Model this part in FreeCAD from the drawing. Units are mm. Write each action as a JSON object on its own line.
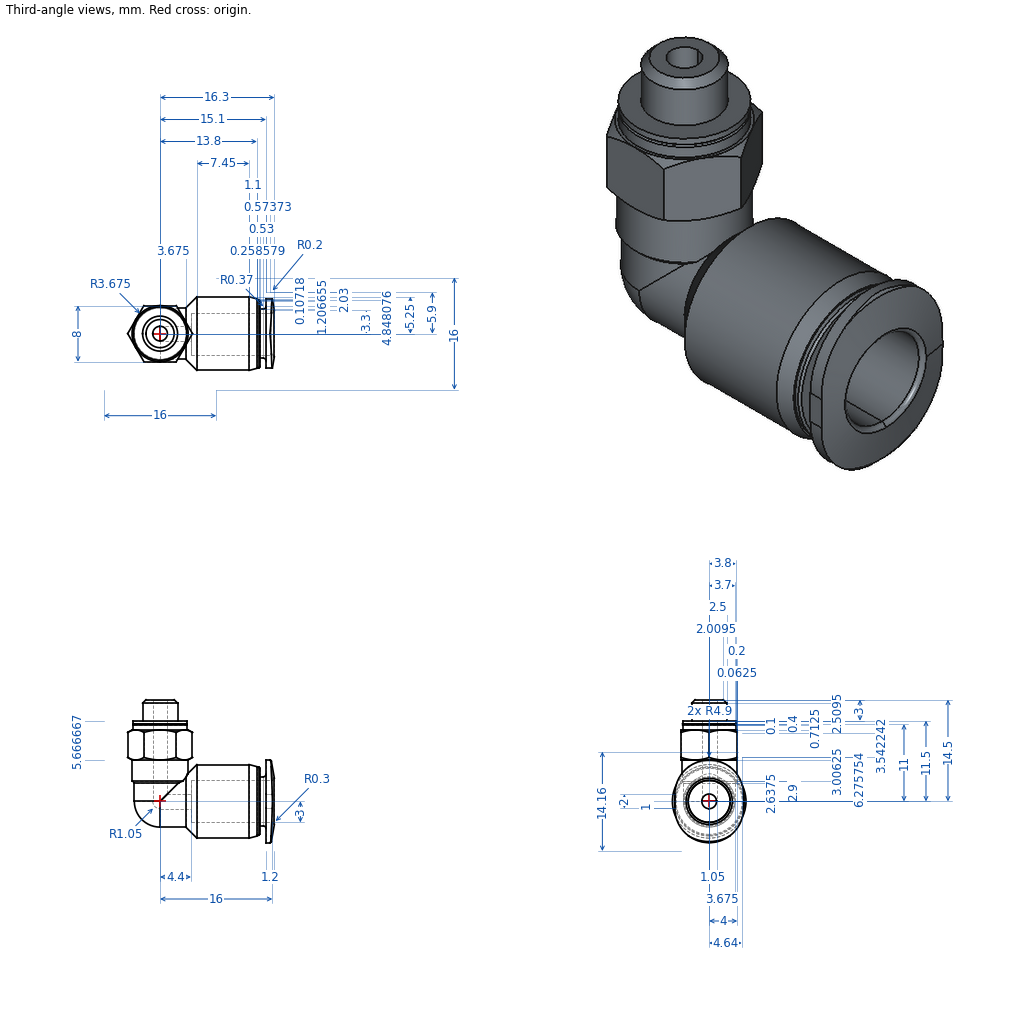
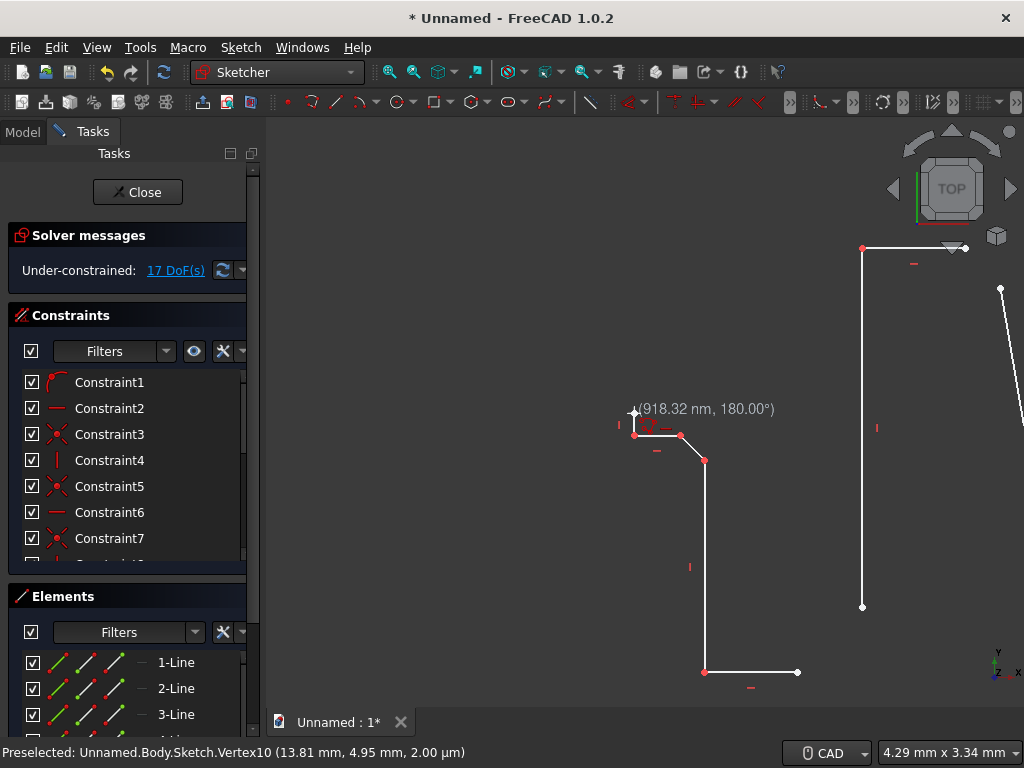
{"action": "scroll", "coordinate": [734, 368], "scroll_direction": "down", "scroll_amount": 11}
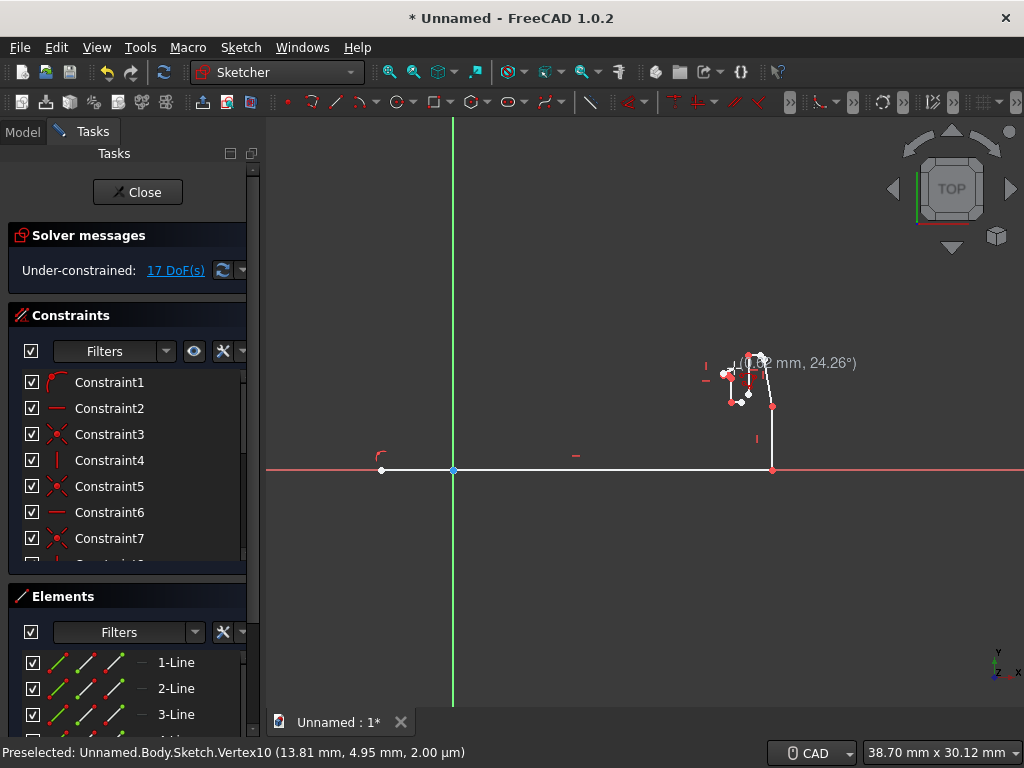
{"action": "left_click", "coordinate": [702, 368]}
{"action": "left_click", "coordinate": [556, 368]}
{"action": "left_click", "coordinate": [525, 398]}
{"action": "left_click", "coordinate": [453, 398]}
{"action": "right_click", "coordinate": [453, 398]}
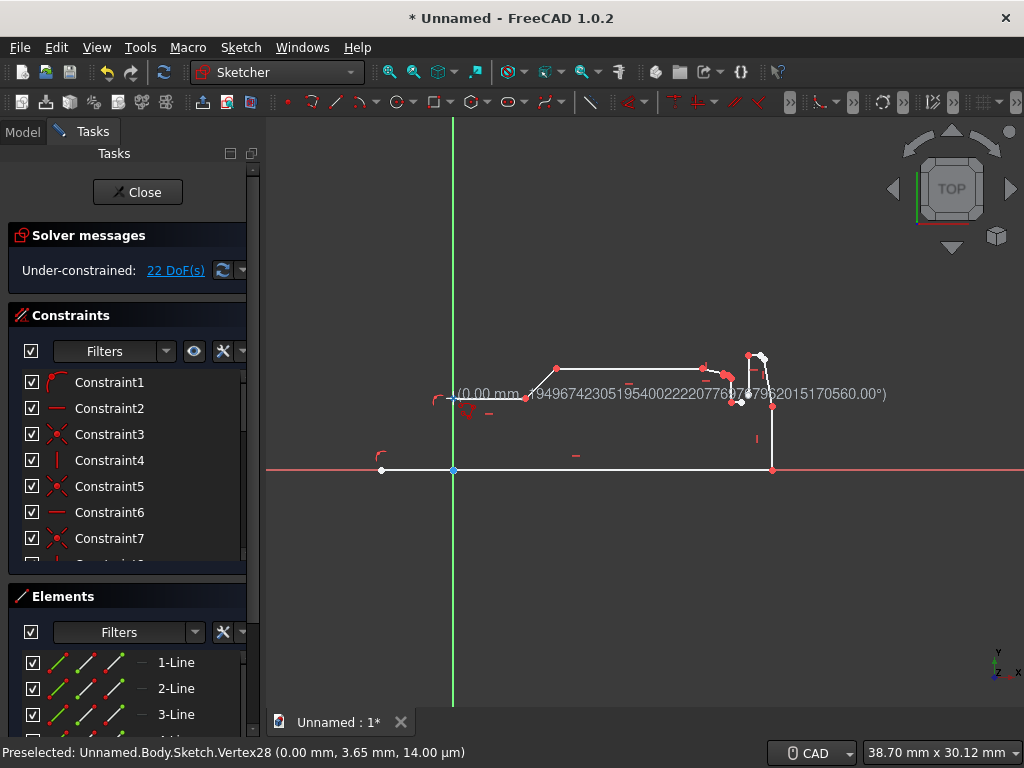
{"action": "key", "text": "g 3 a"}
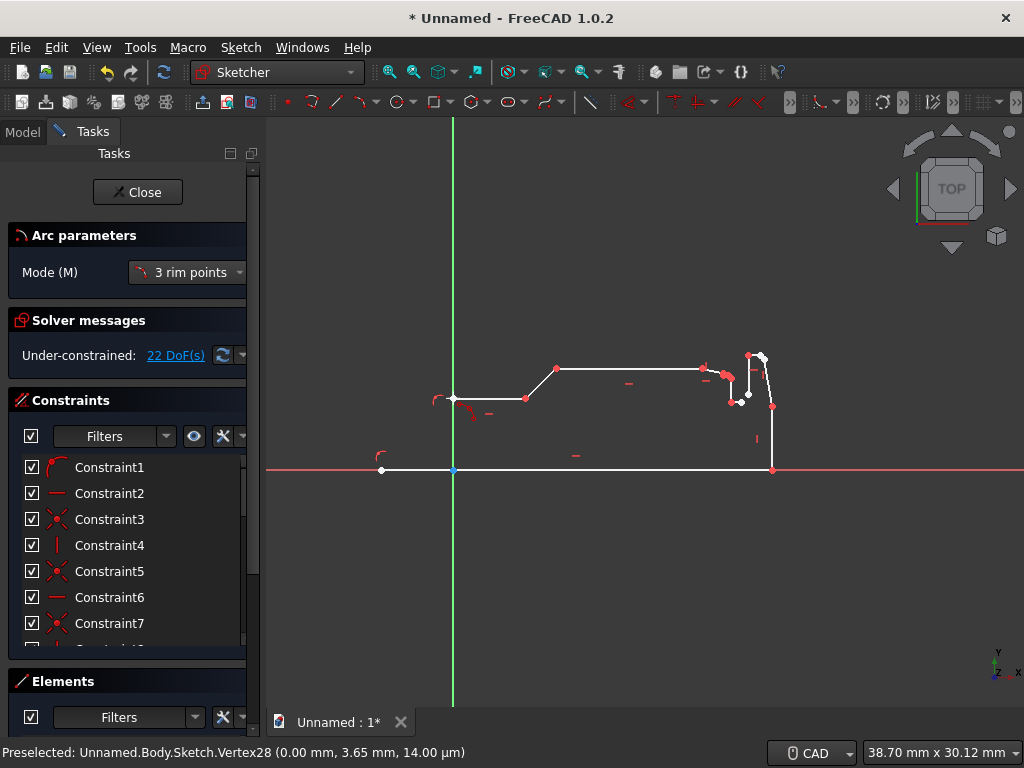
{"action": "scroll", "coordinate": [764, 358], "scroll_direction": "up", "scroll_amount": 6}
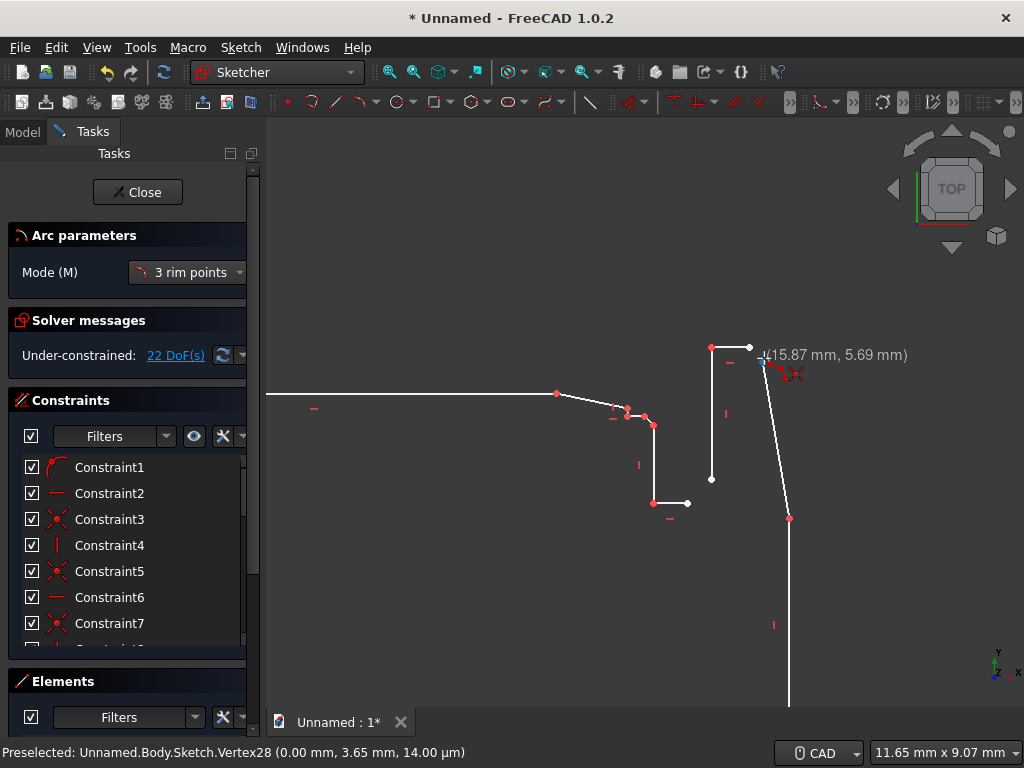
{"action": "left_click", "coordinate": [763, 362]}
{"action": "left_click", "coordinate": [750, 347]}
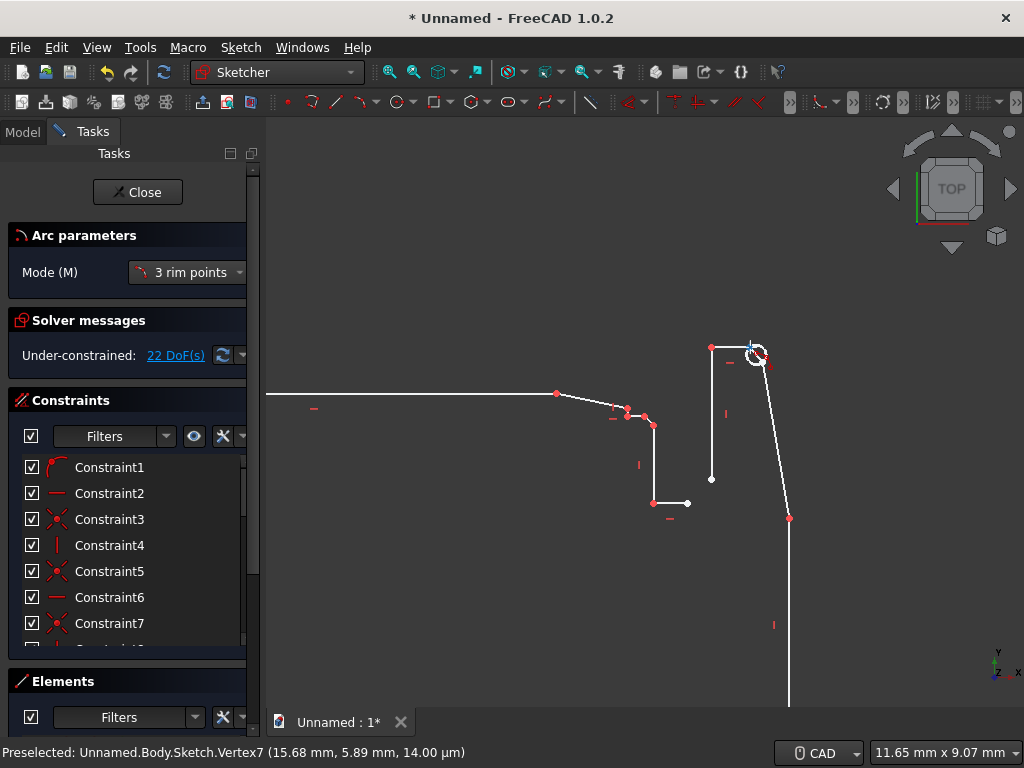
{"action": "scroll", "coordinate": [758, 350], "scroll_direction": "up", "scroll_amount": 9}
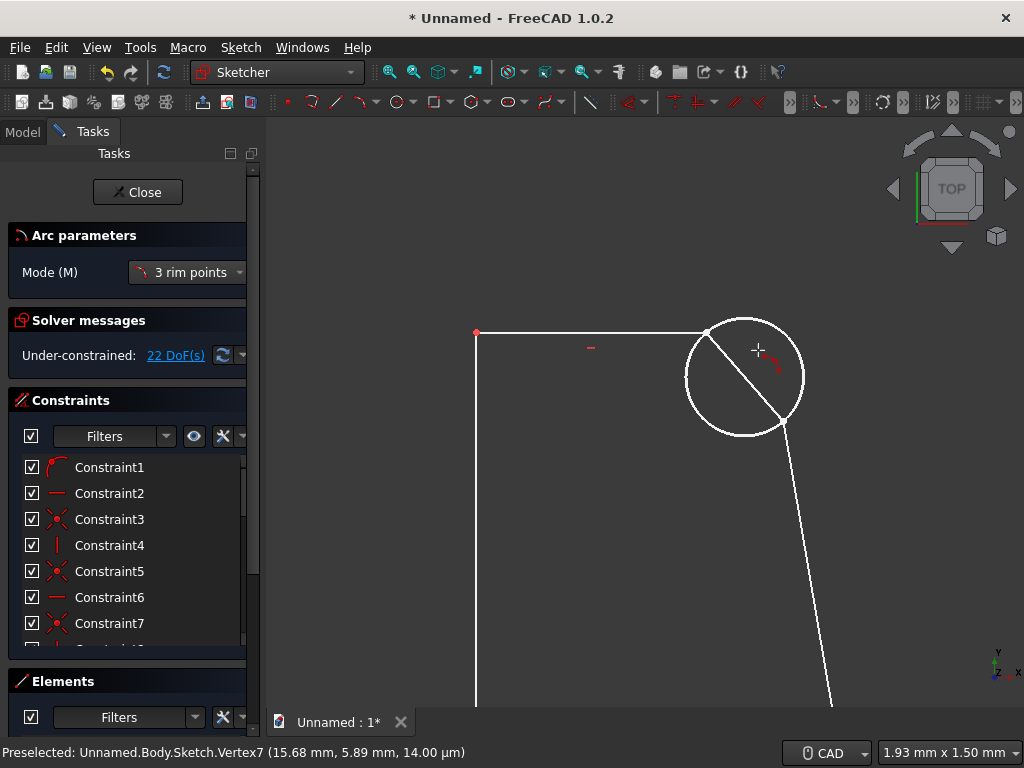
{"action": "left_click", "coordinate": [754, 347]}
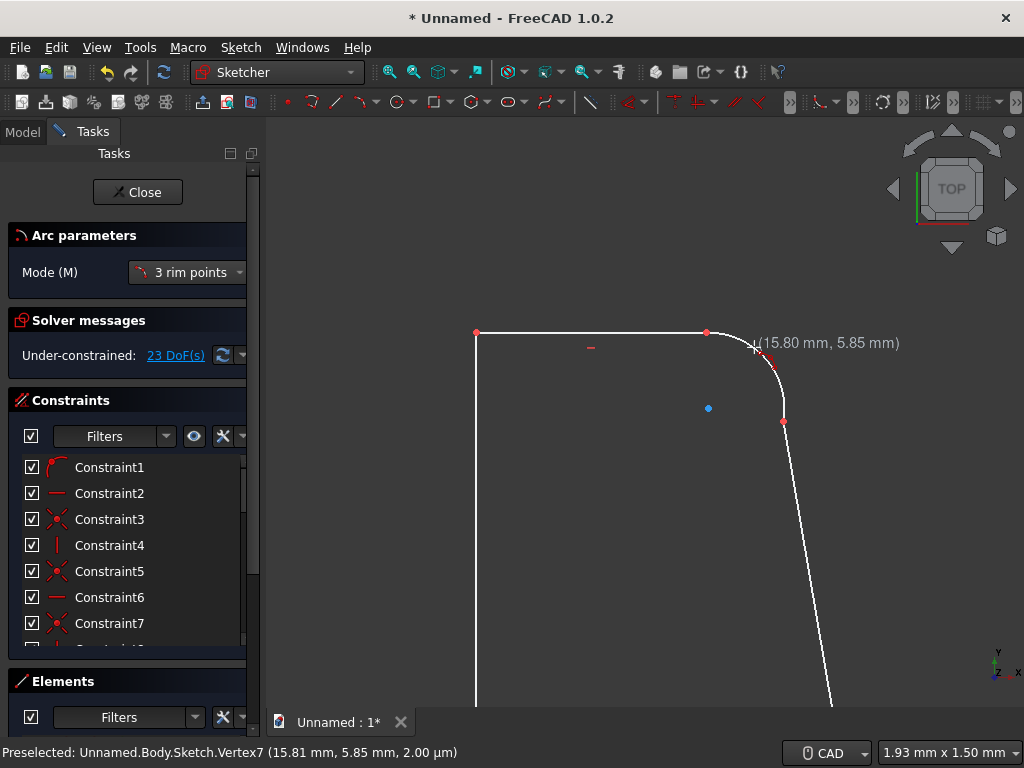
{"action": "scroll", "coordinate": [763, 356], "scroll_direction": "down", "scroll_amount": 15}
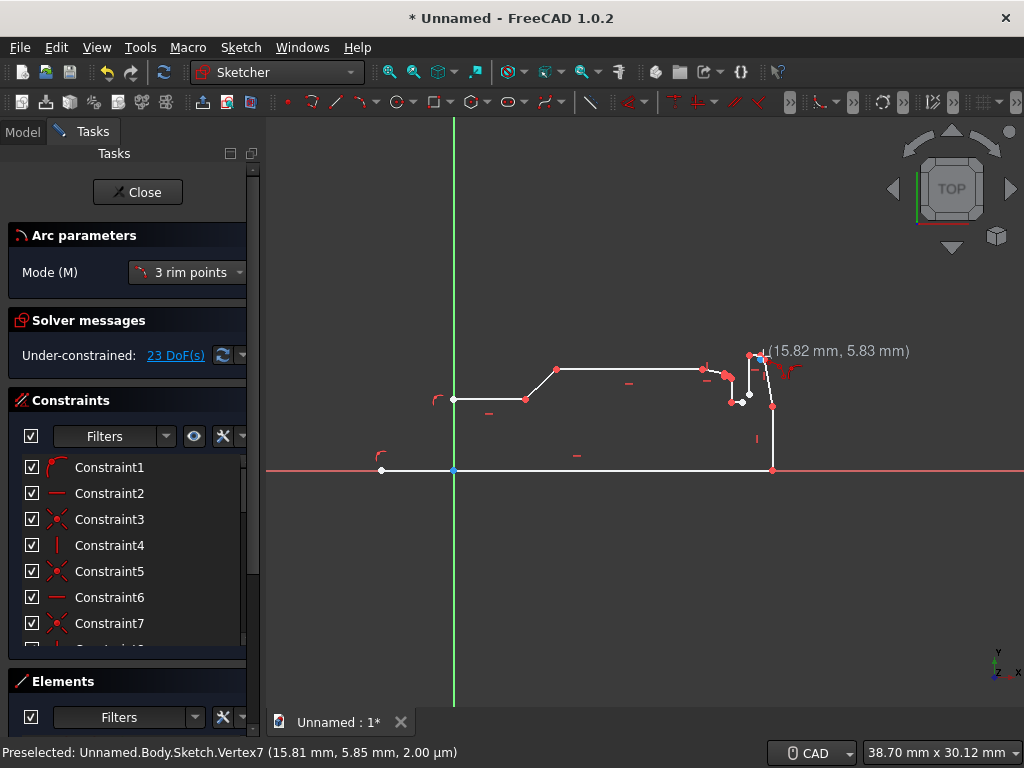
{"action": "scroll", "coordinate": [749, 395], "scroll_direction": "up", "scroll_amount": 3}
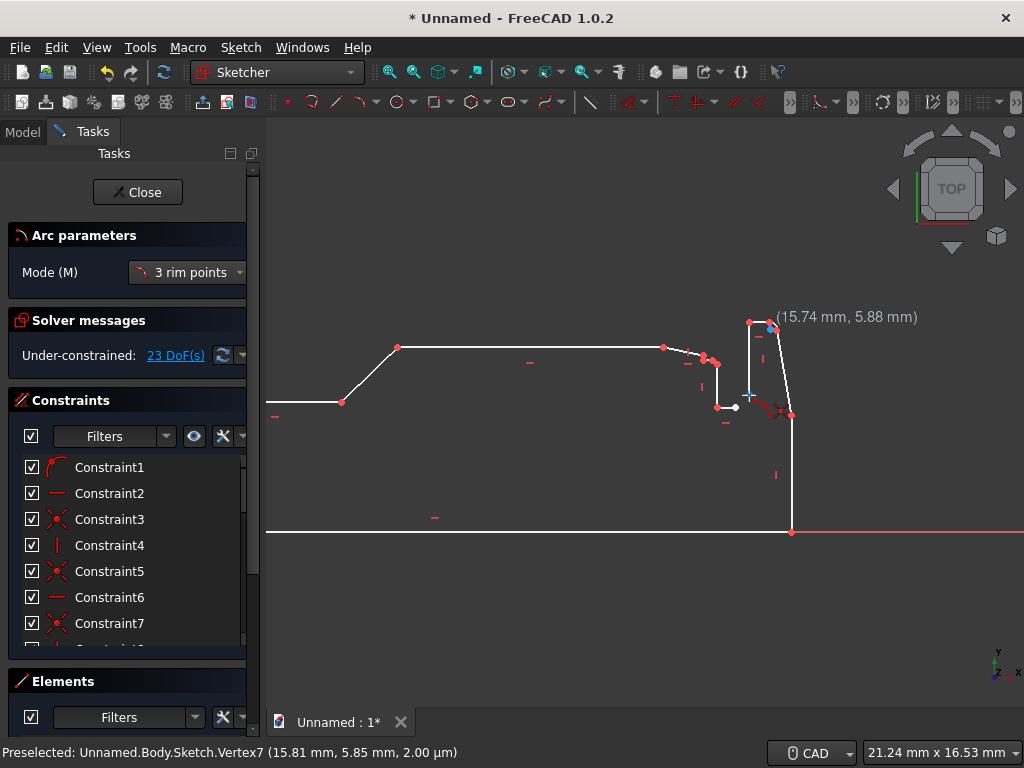
{"action": "left_click", "coordinate": [749, 395]}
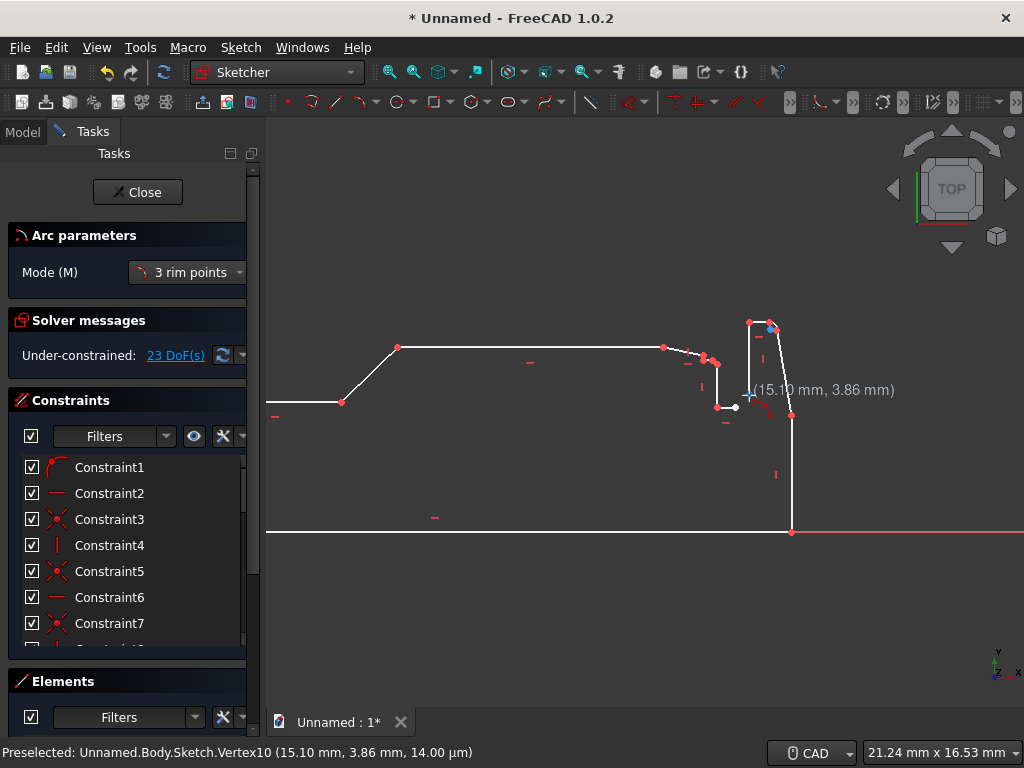
{"action": "scroll", "coordinate": [736, 407], "scroll_direction": "up", "scroll_amount": 3}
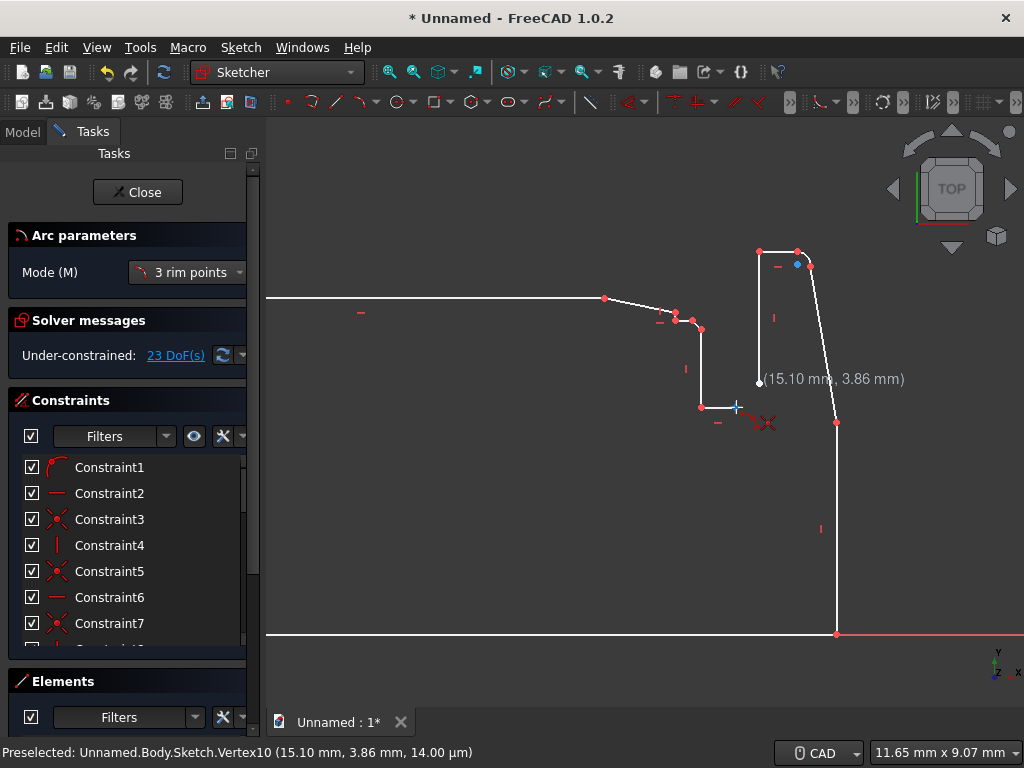
{"action": "left_click", "coordinate": [735, 408]}